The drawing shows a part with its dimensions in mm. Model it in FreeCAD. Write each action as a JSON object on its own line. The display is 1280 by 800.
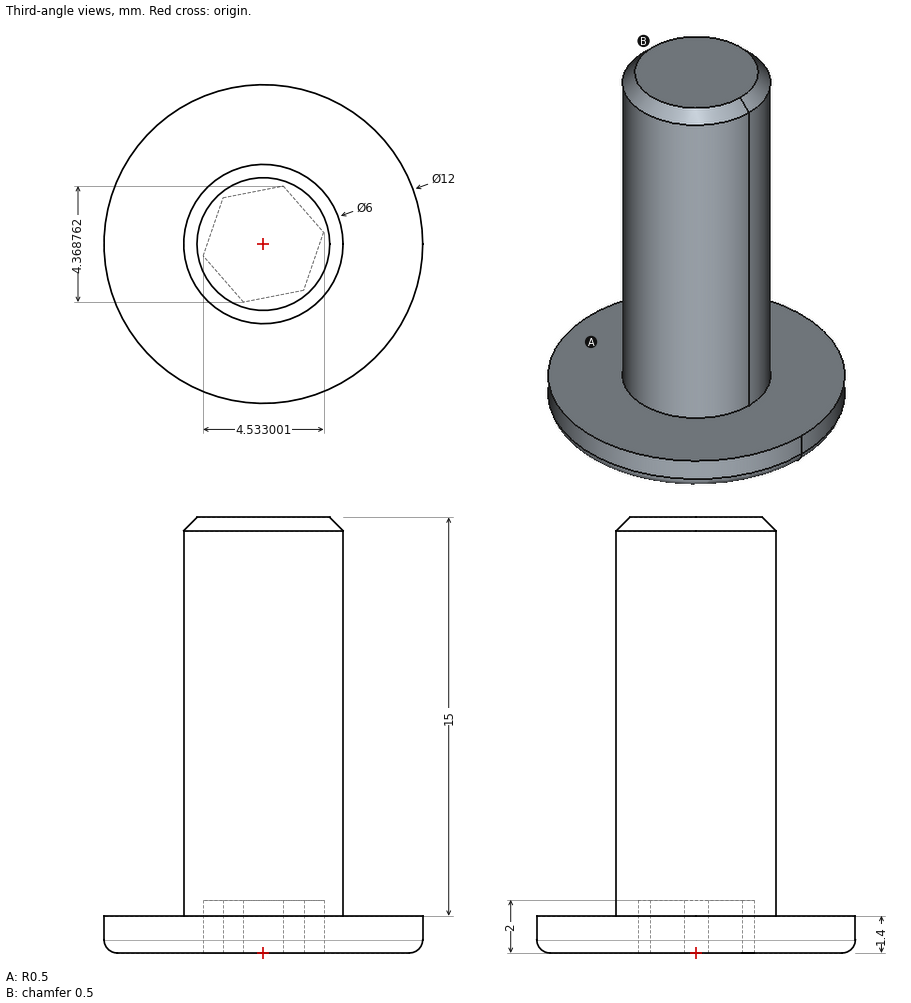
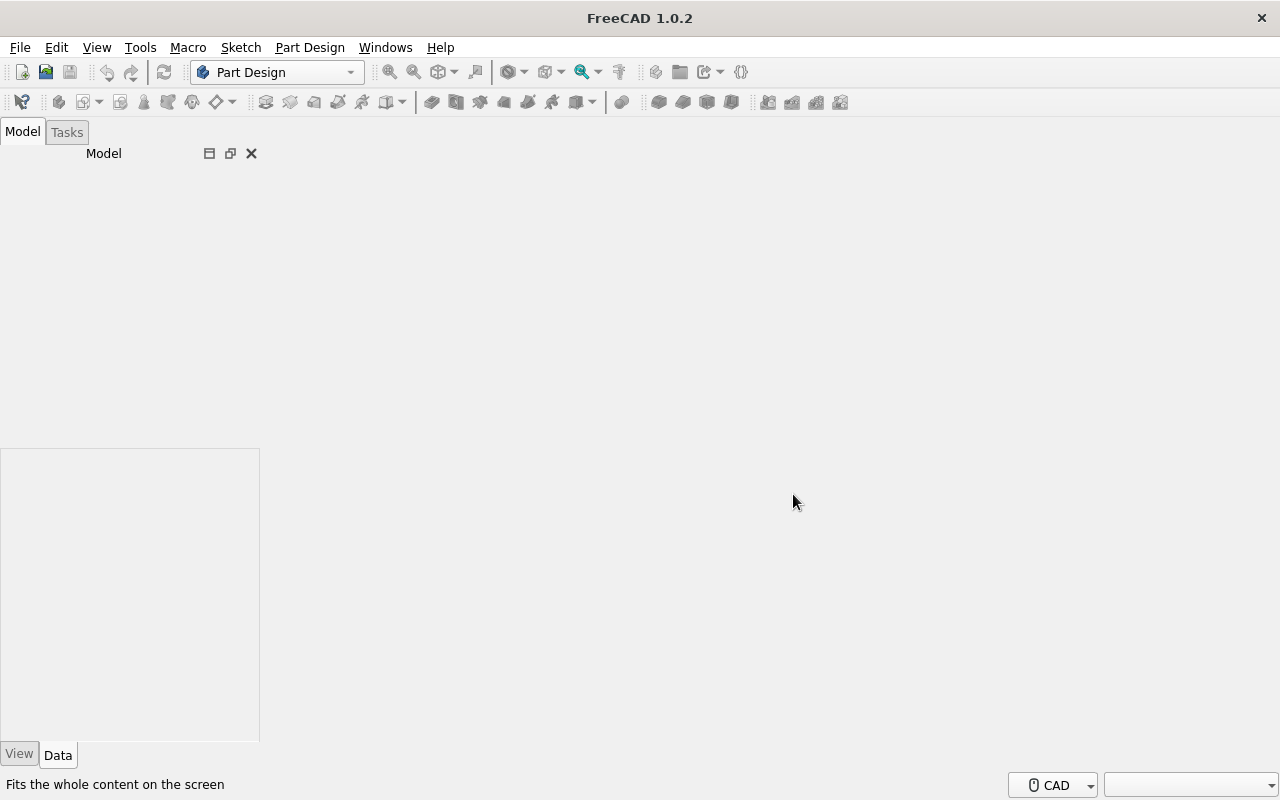
{"action": "left_click", "coordinate": [22, 72]}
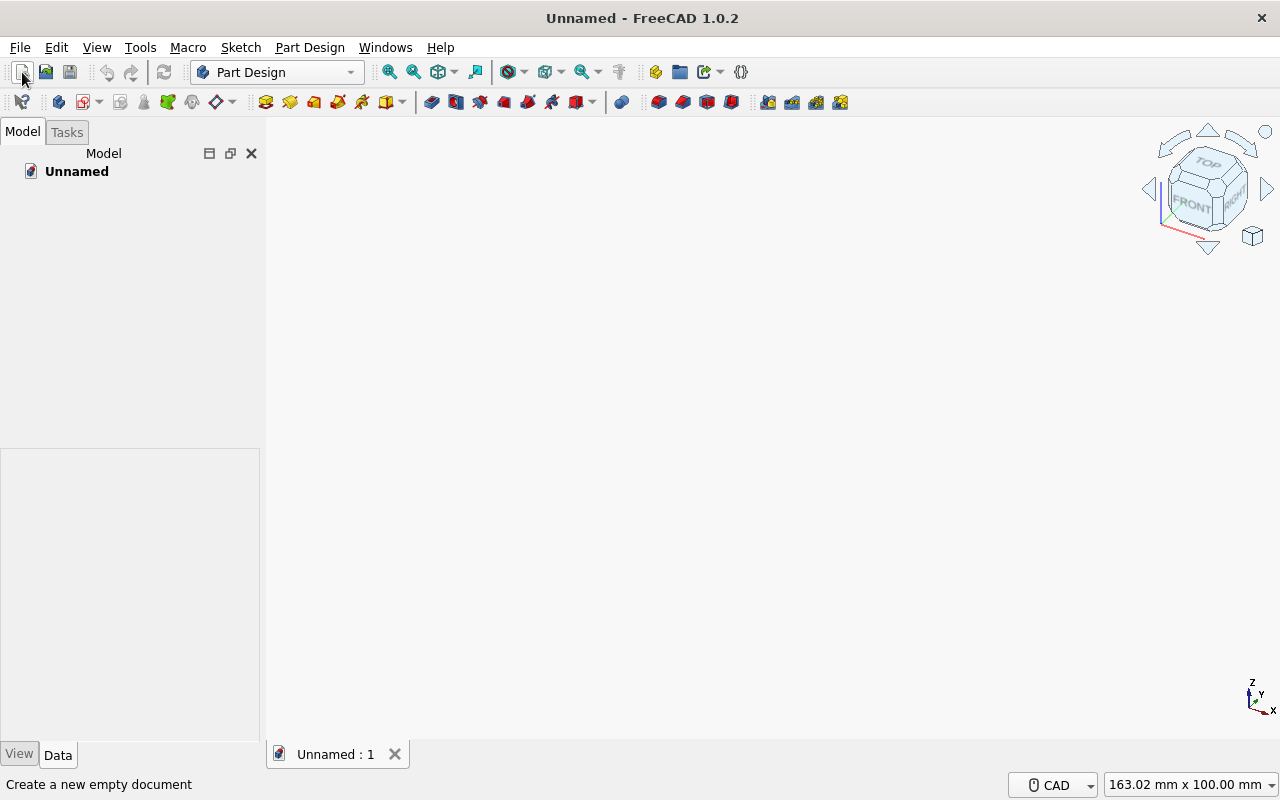
{"action": "left_click", "coordinate": [84, 102]}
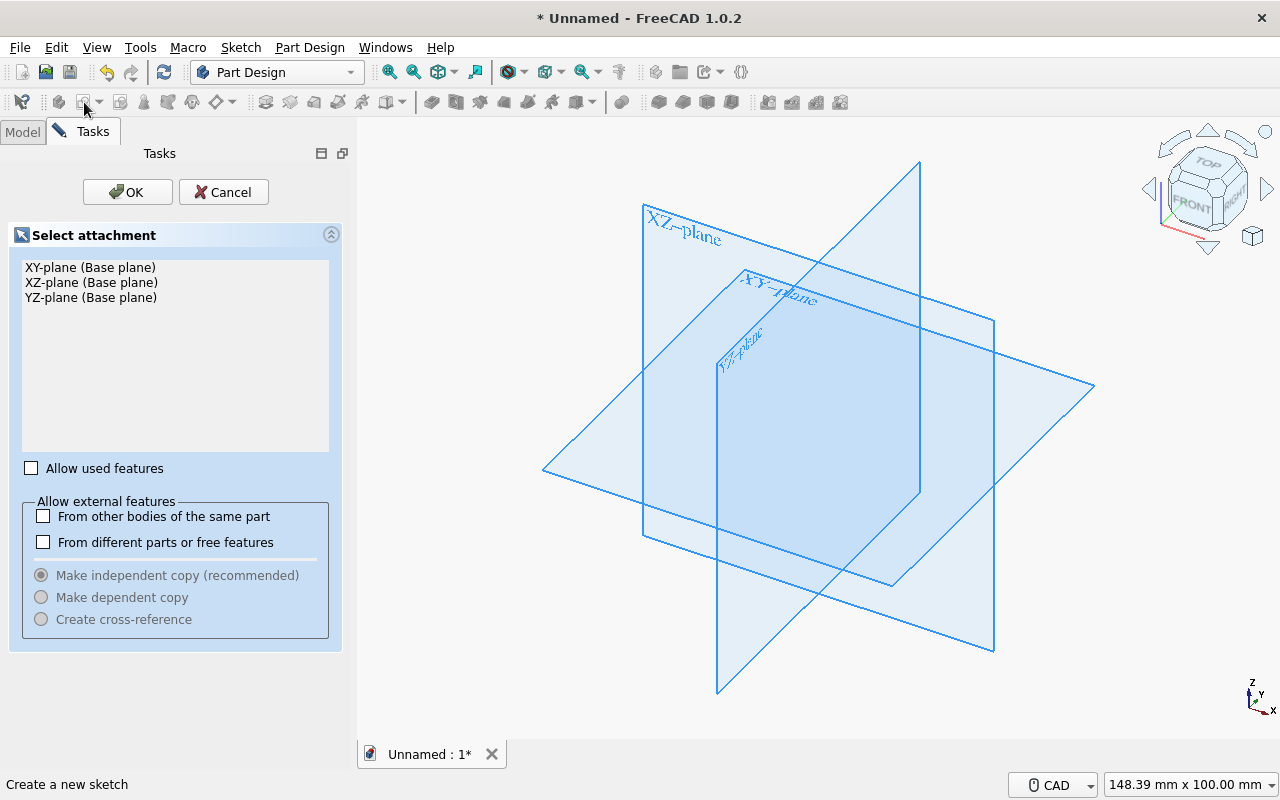
{"action": "left_click", "coordinate": [82, 268]}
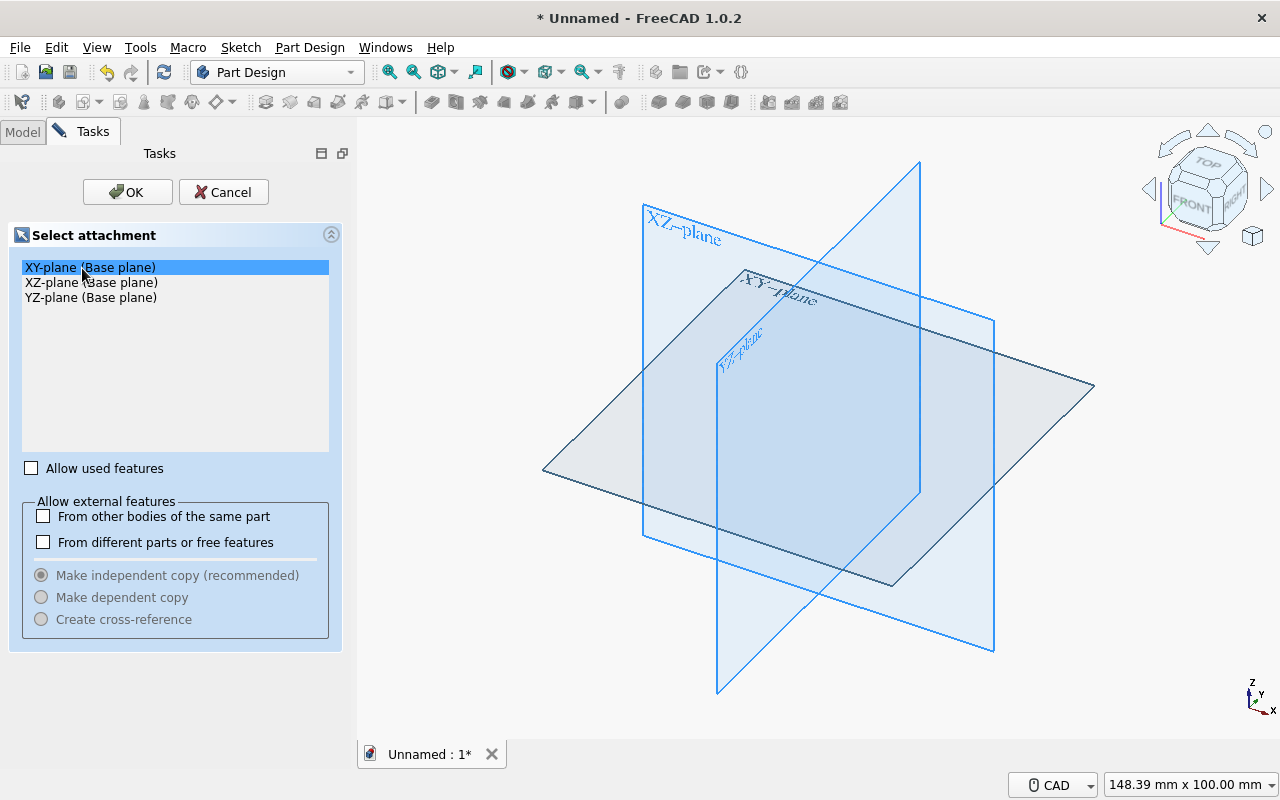
{"action": "left_click", "coordinate": [128, 192]}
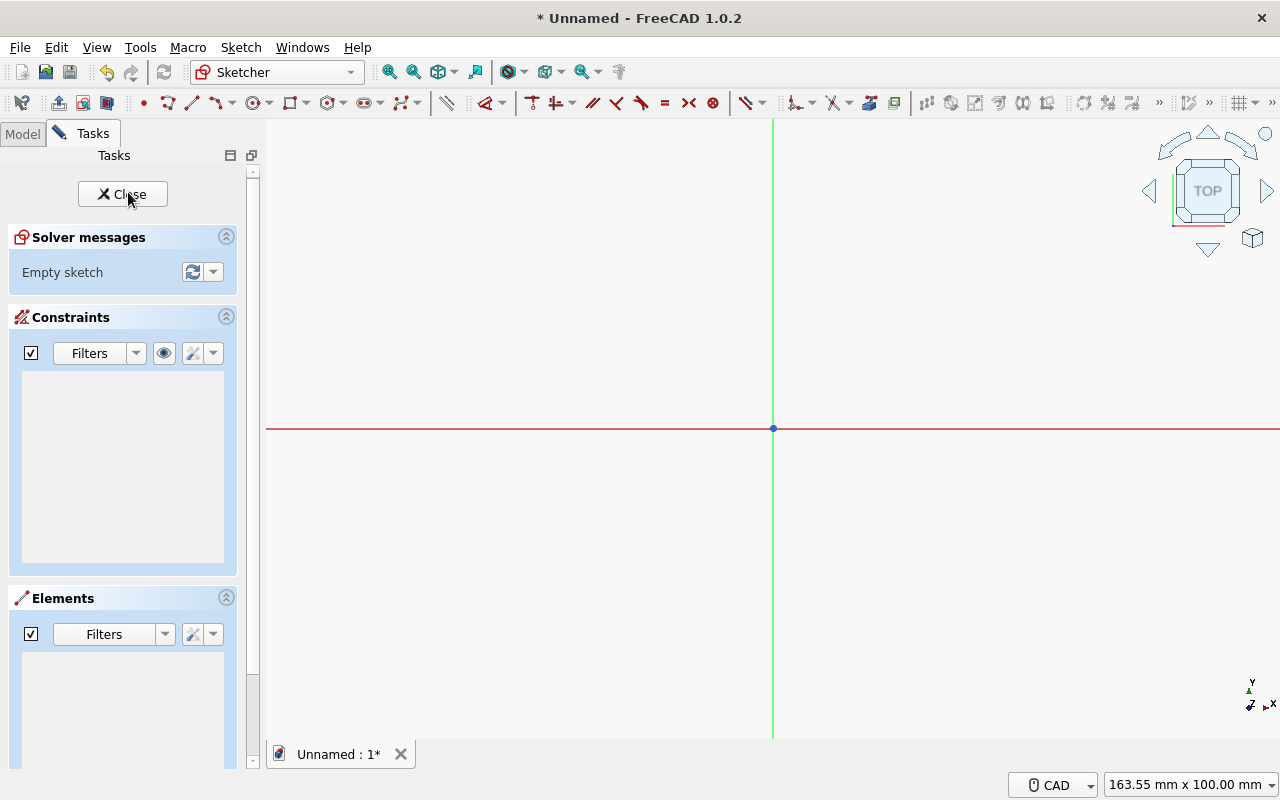
{"action": "scroll", "coordinate": [790, 429], "scroll_direction": "up", "scroll_amount": 8}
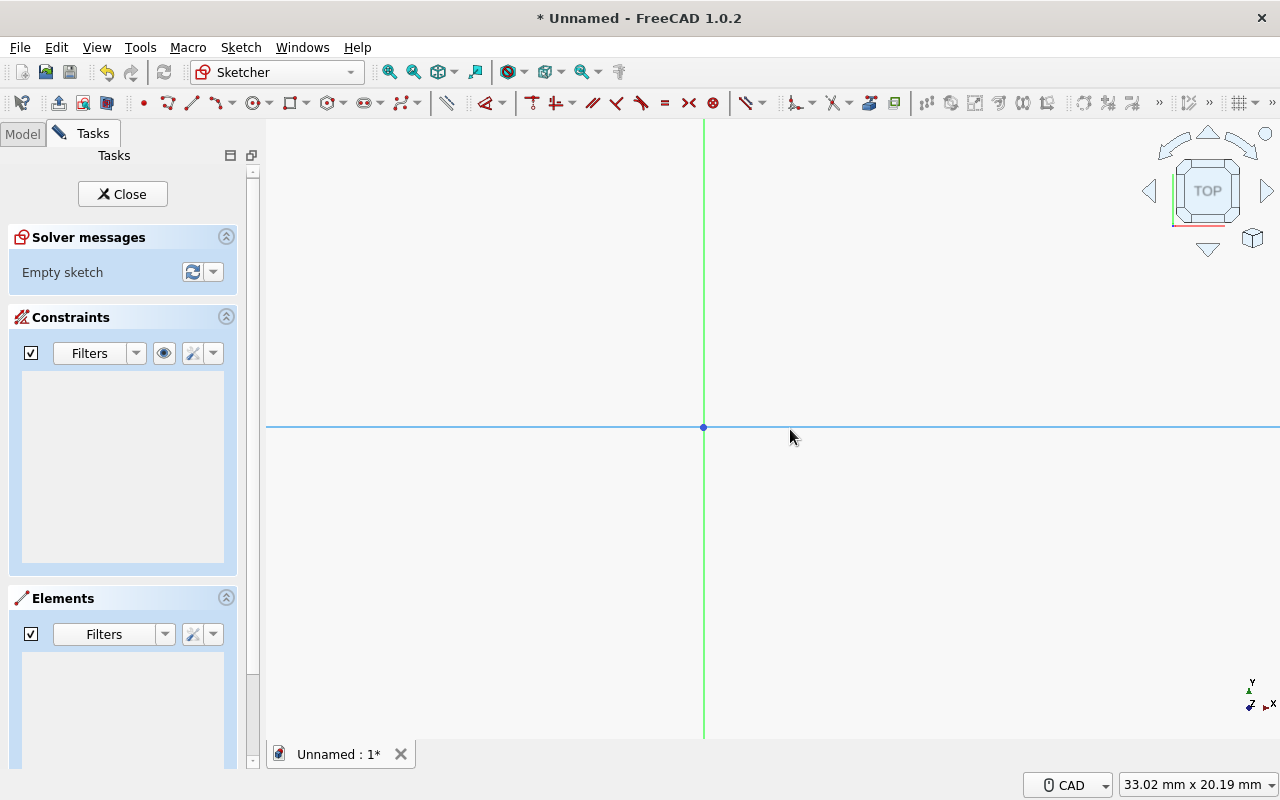
{"action": "left_click", "coordinate": [254, 104]}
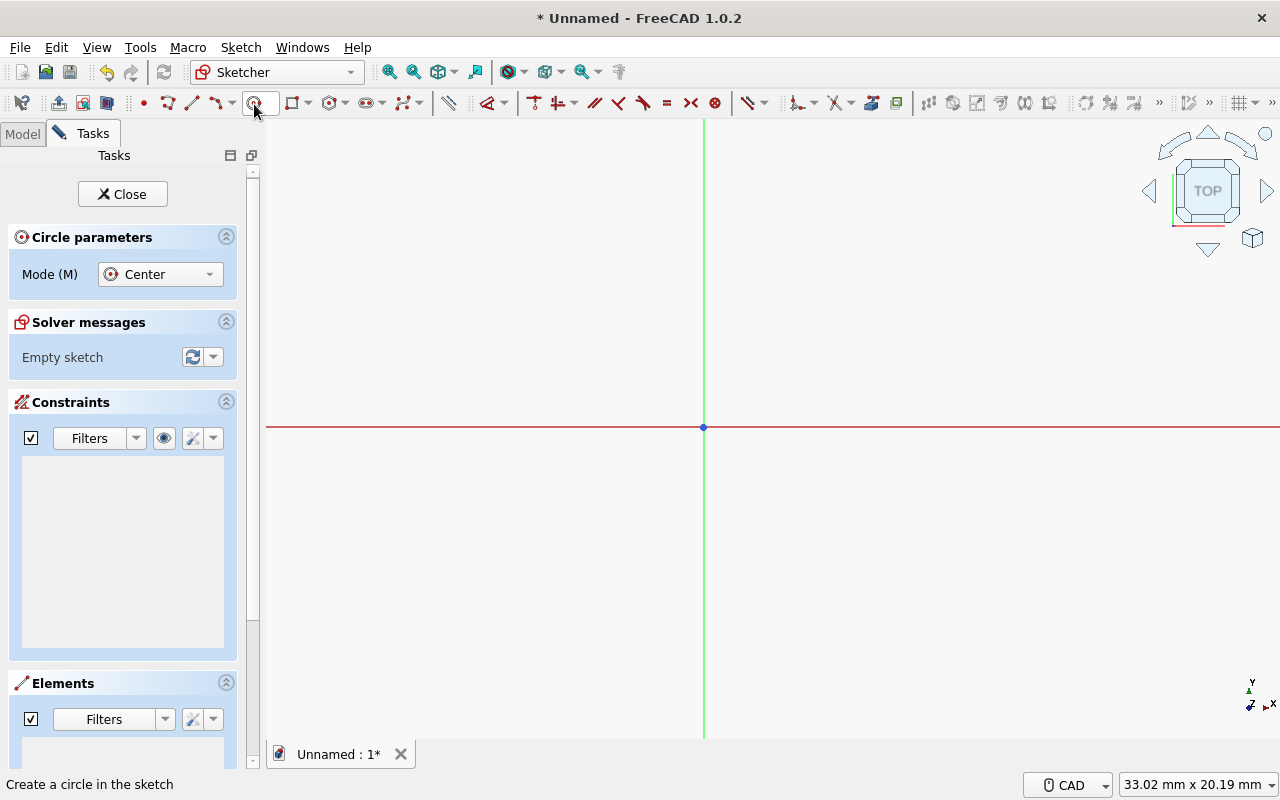
{"action": "left_click", "coordinate": [704, 427]}
{"action": "mouse_move", "coordinate": [834, 297]}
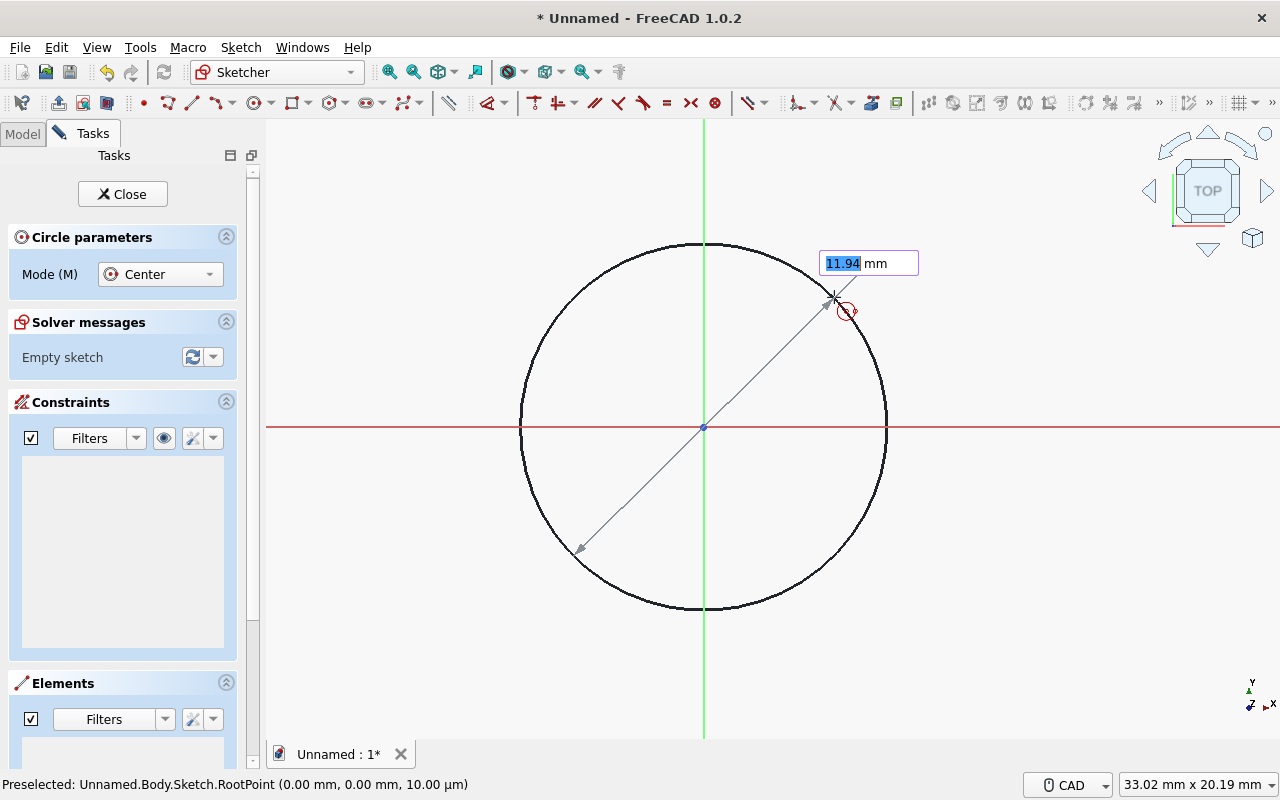
{"action": "type", "text": "12"}
{"action": "key", "text": "Return"}
{"action": "key", "text": "Escape"}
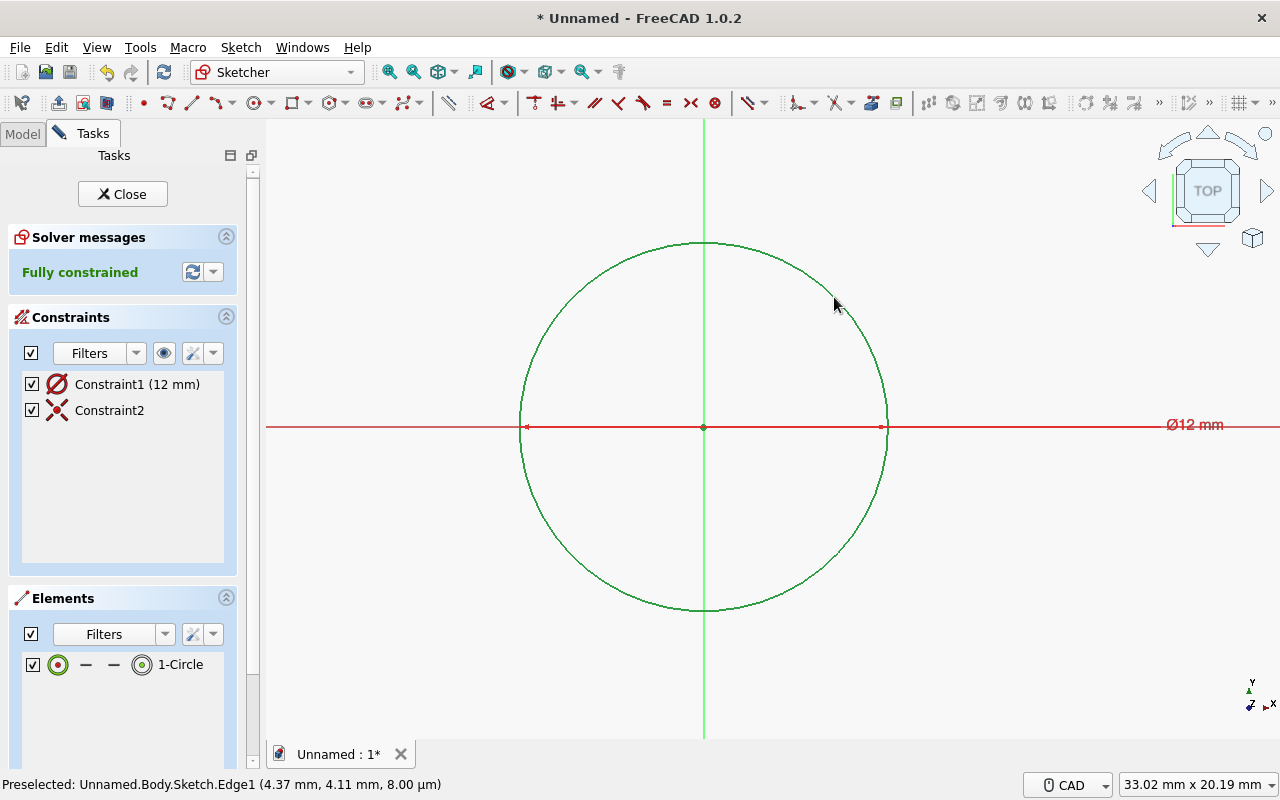
{"action": "left_click", "coordinate": [123, 194]}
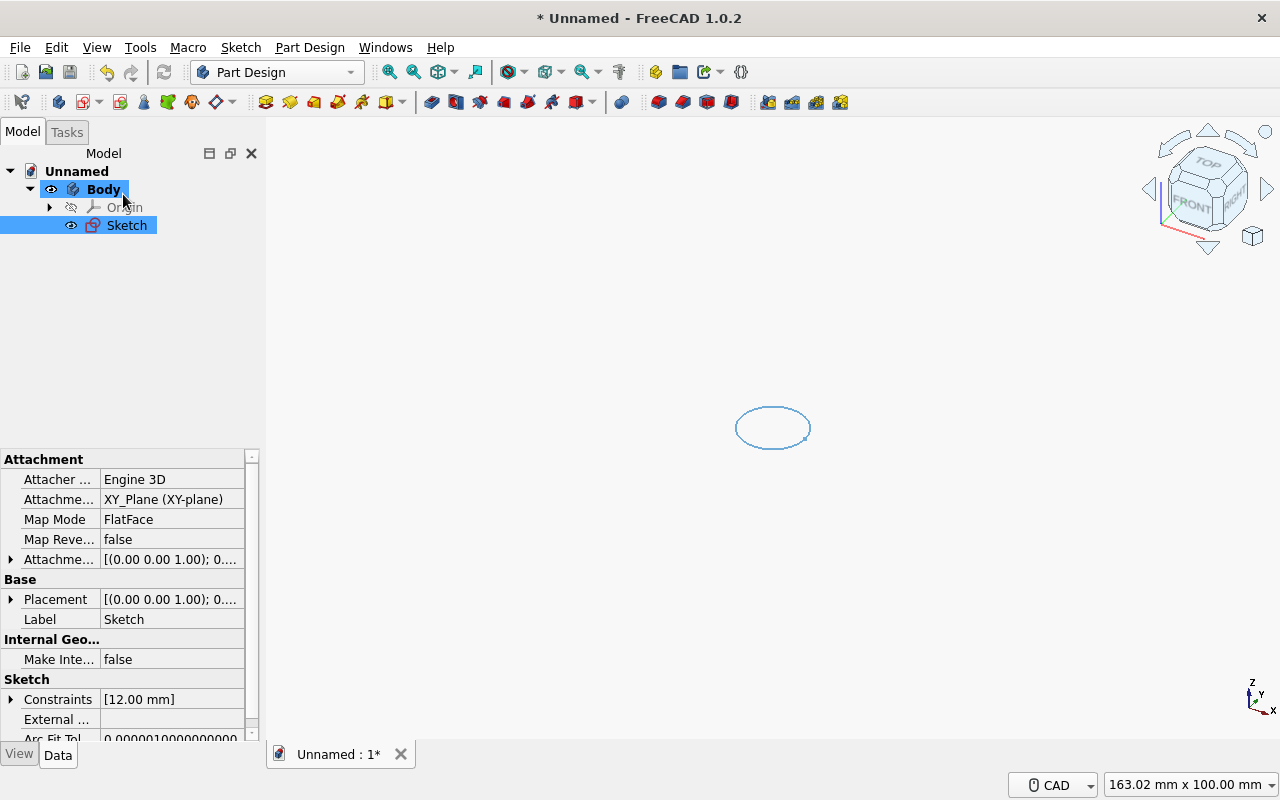
{"action": "left_click", "coordinate": [266, 102]}